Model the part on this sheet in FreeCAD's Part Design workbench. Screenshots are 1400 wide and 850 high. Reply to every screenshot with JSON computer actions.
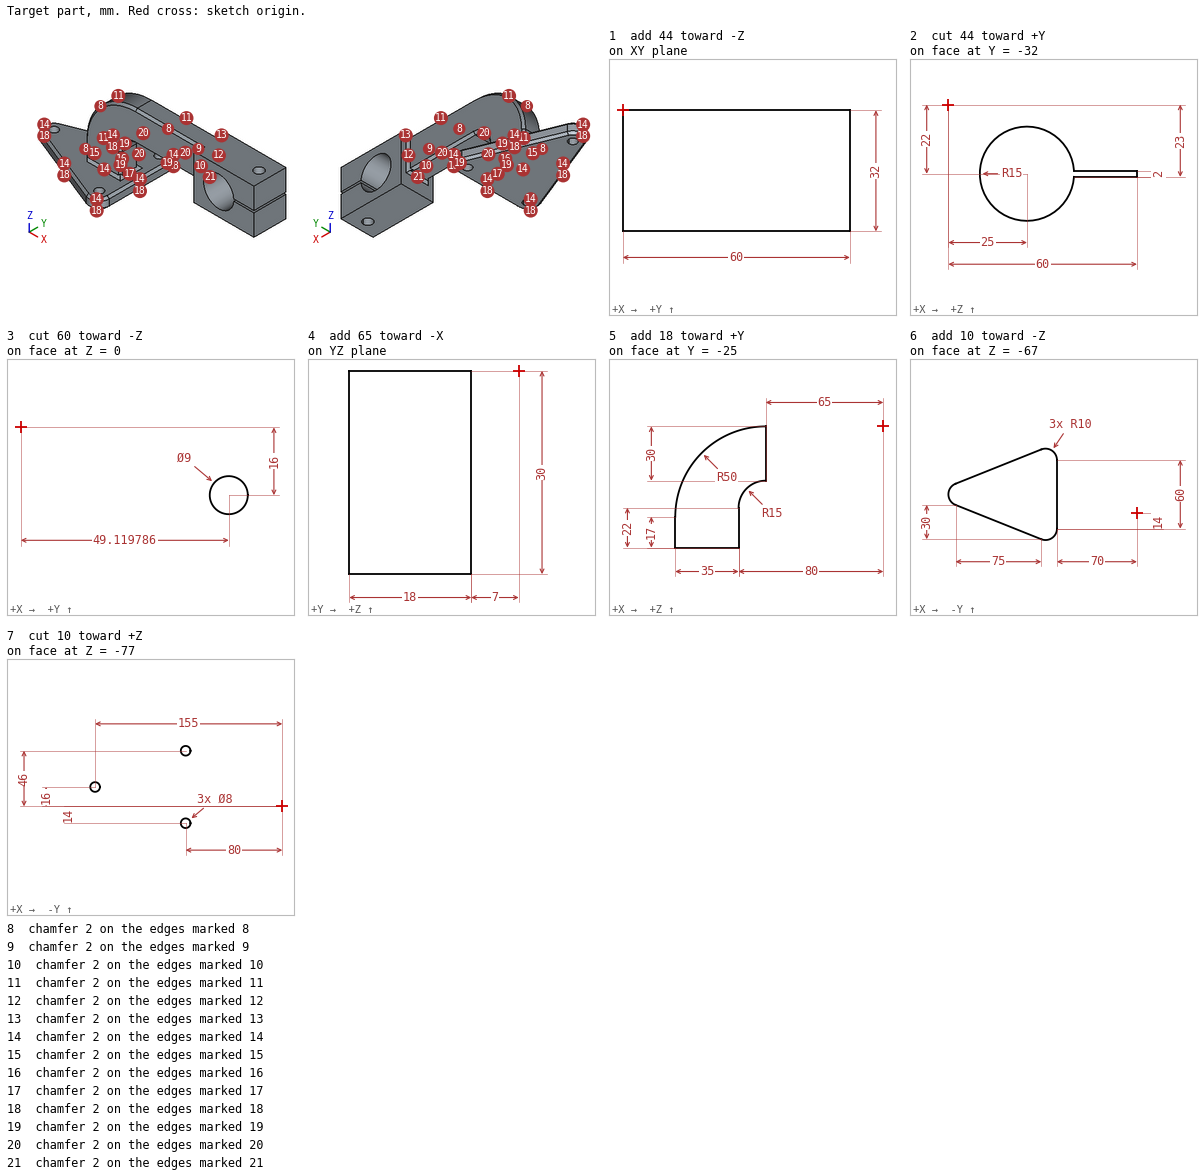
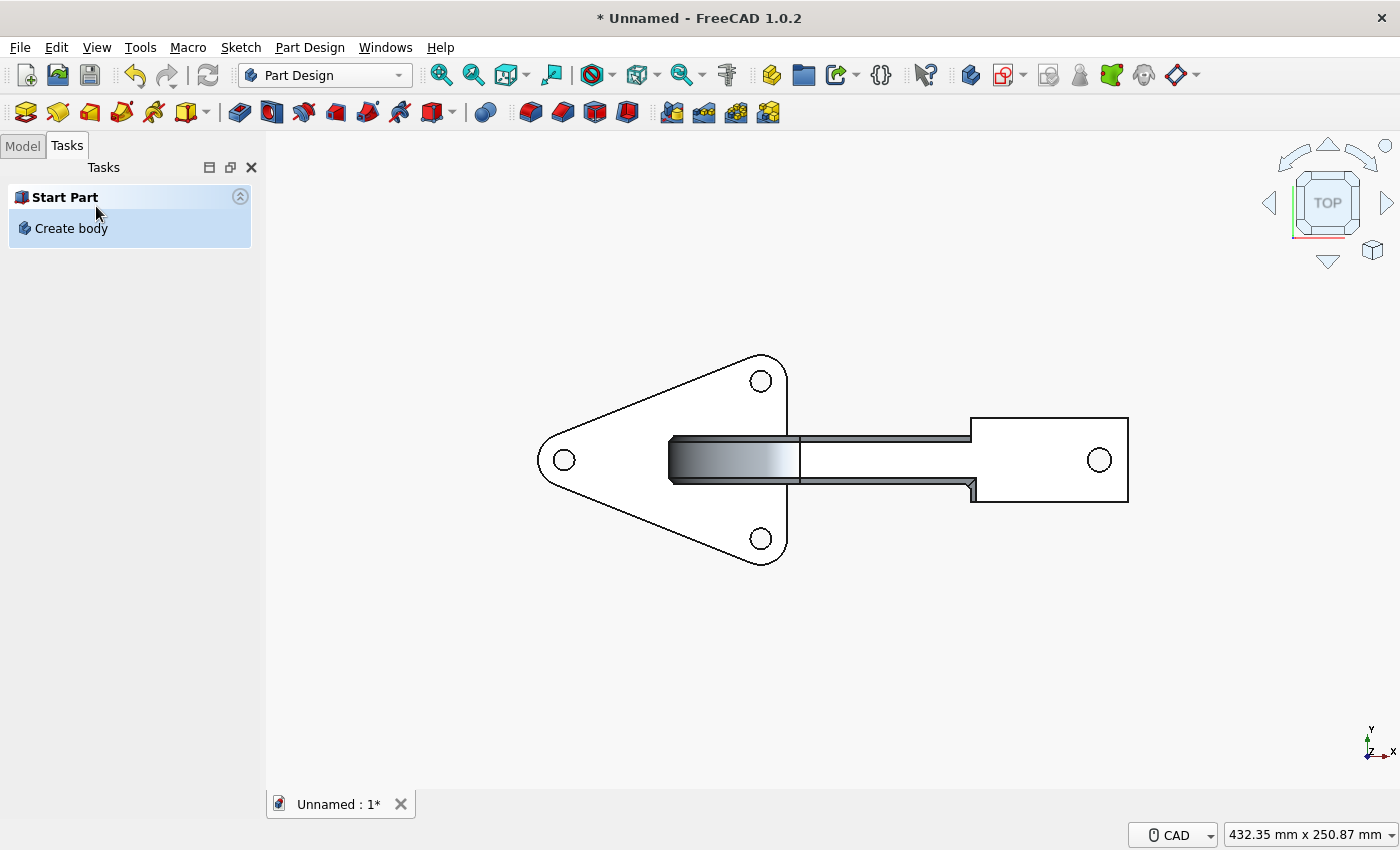
{"action": "key", "text": "1"}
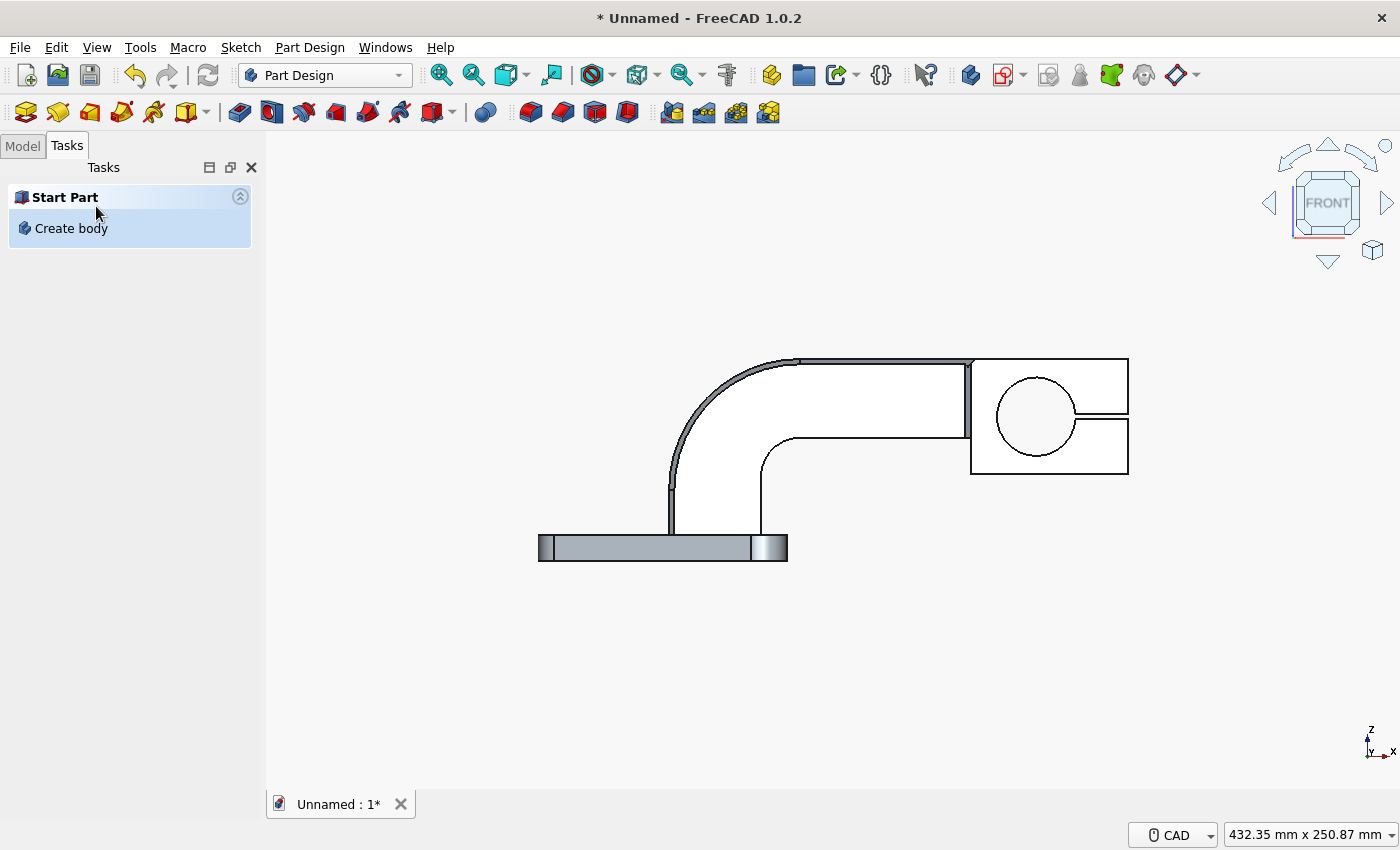
{"action": "key", "text": "3"}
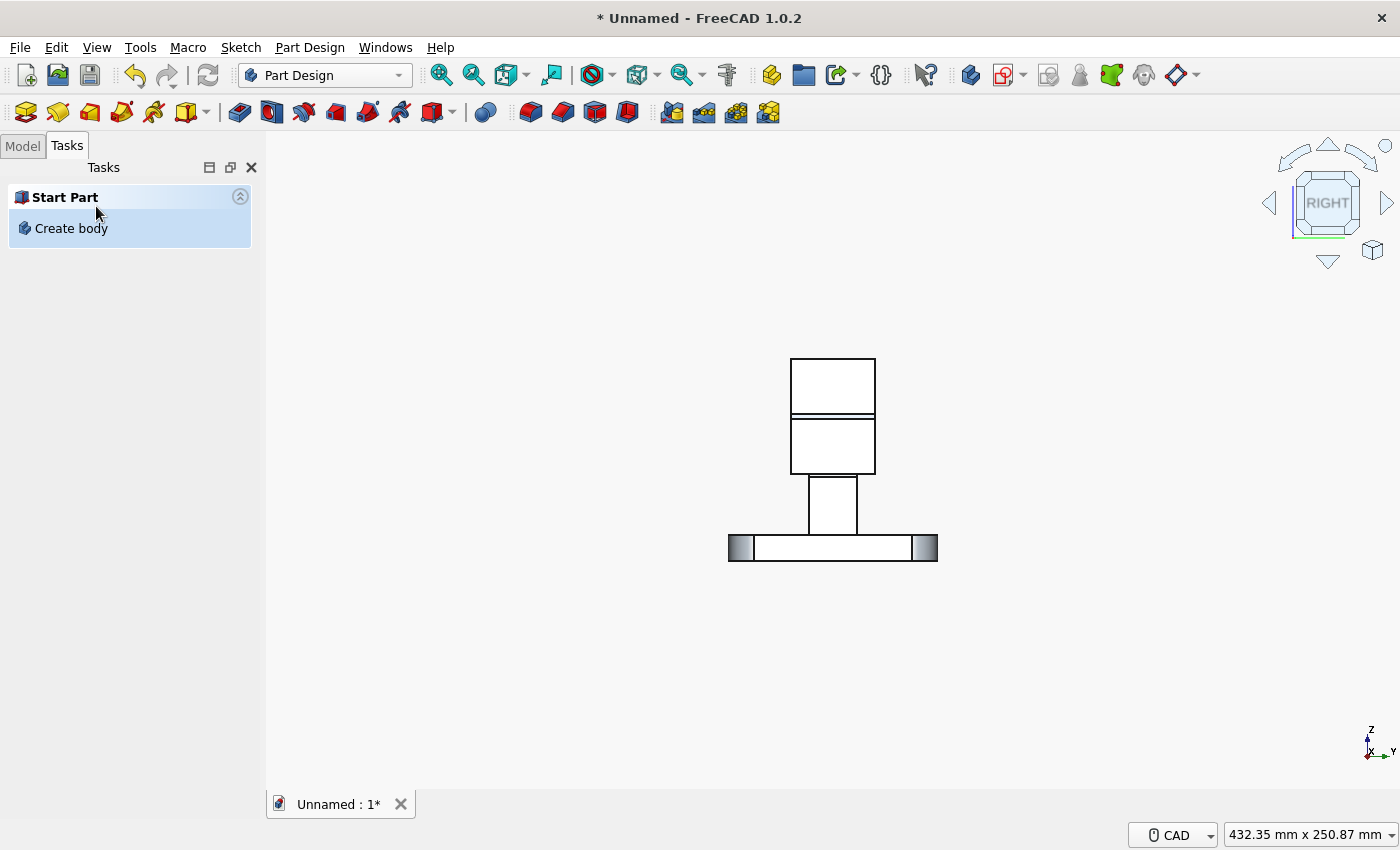
{"action": "left_click", "coordinate": [442, 76]}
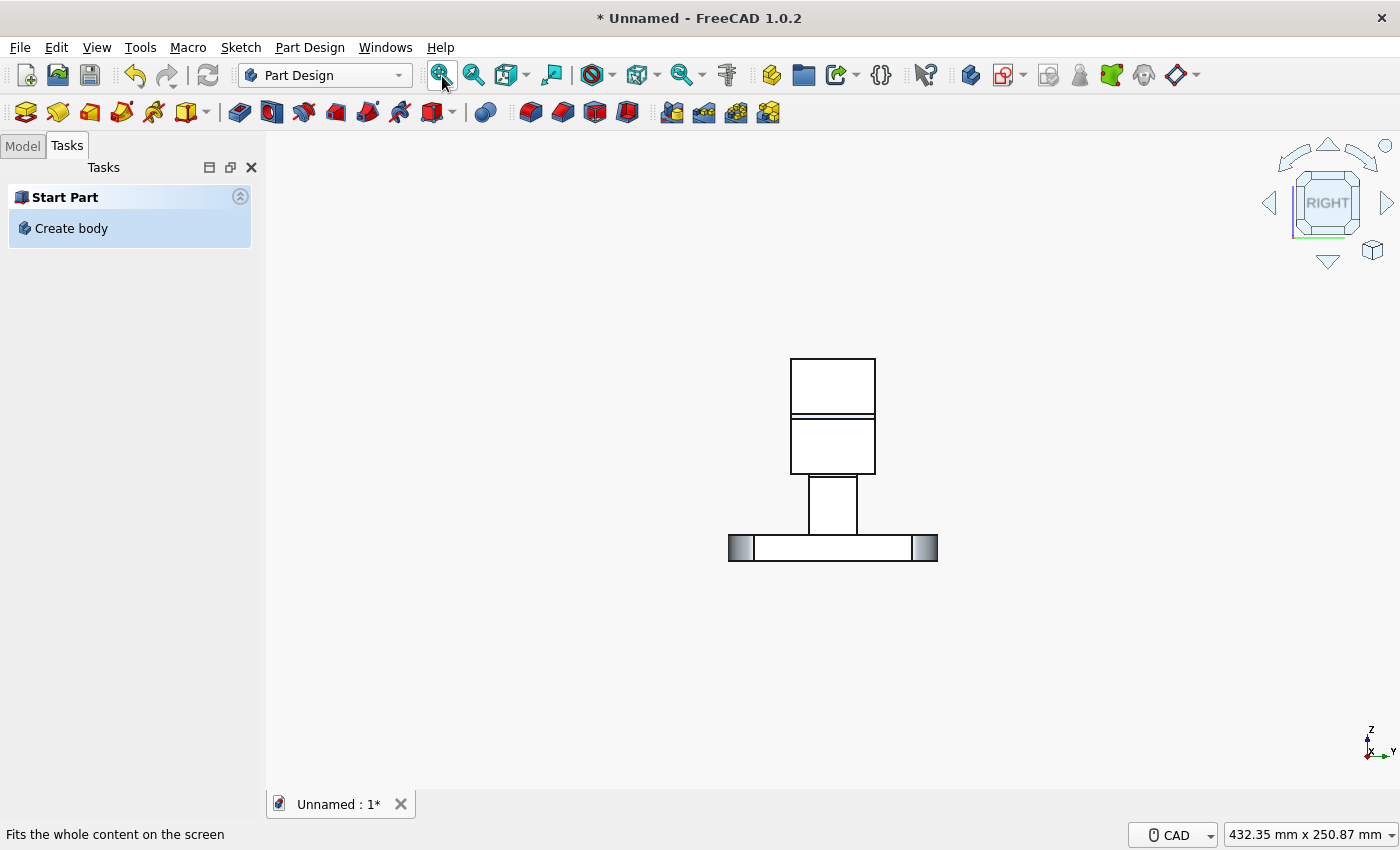
{"action": "key", "text": "5"}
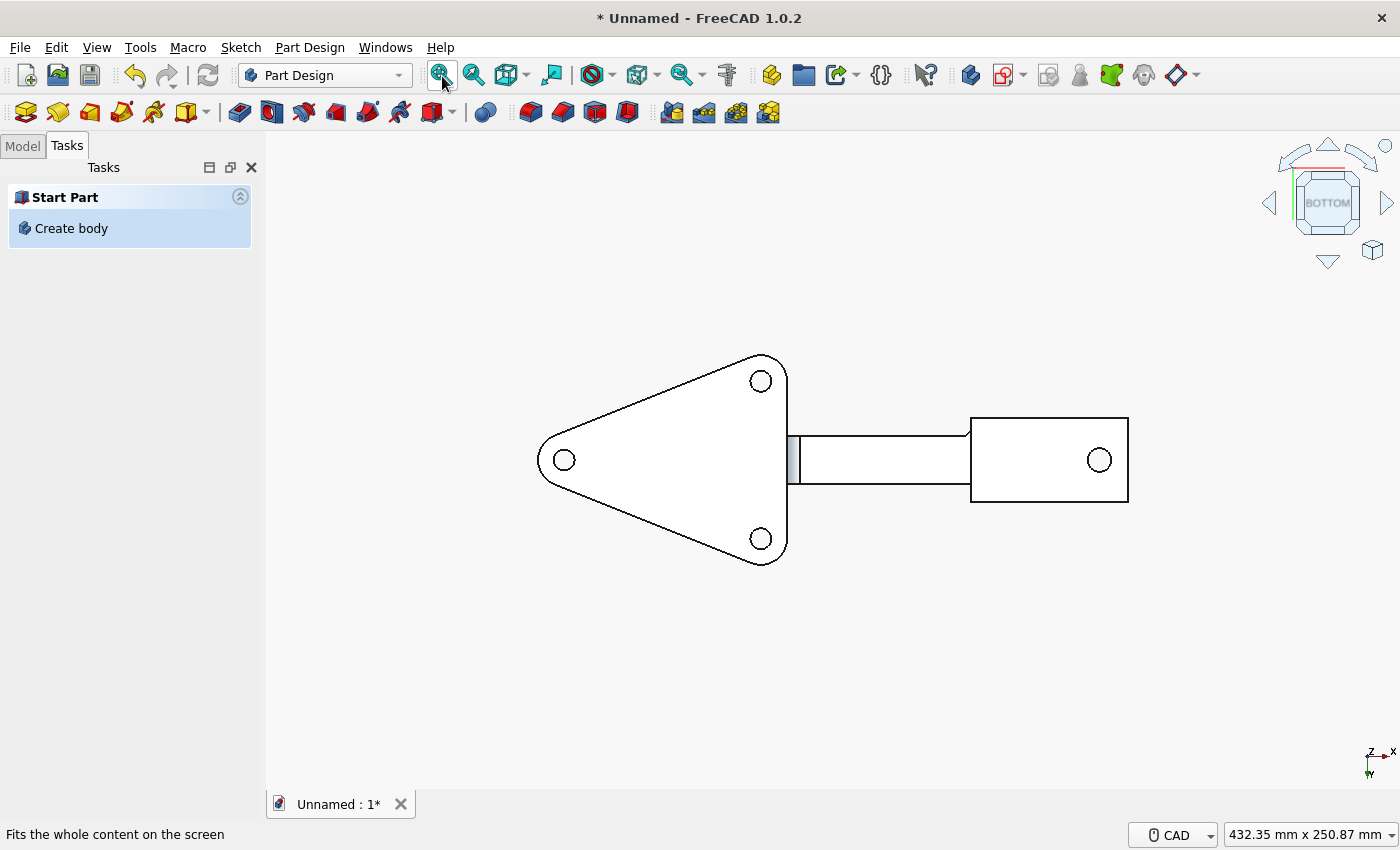
{"action": "key", "text": "4"}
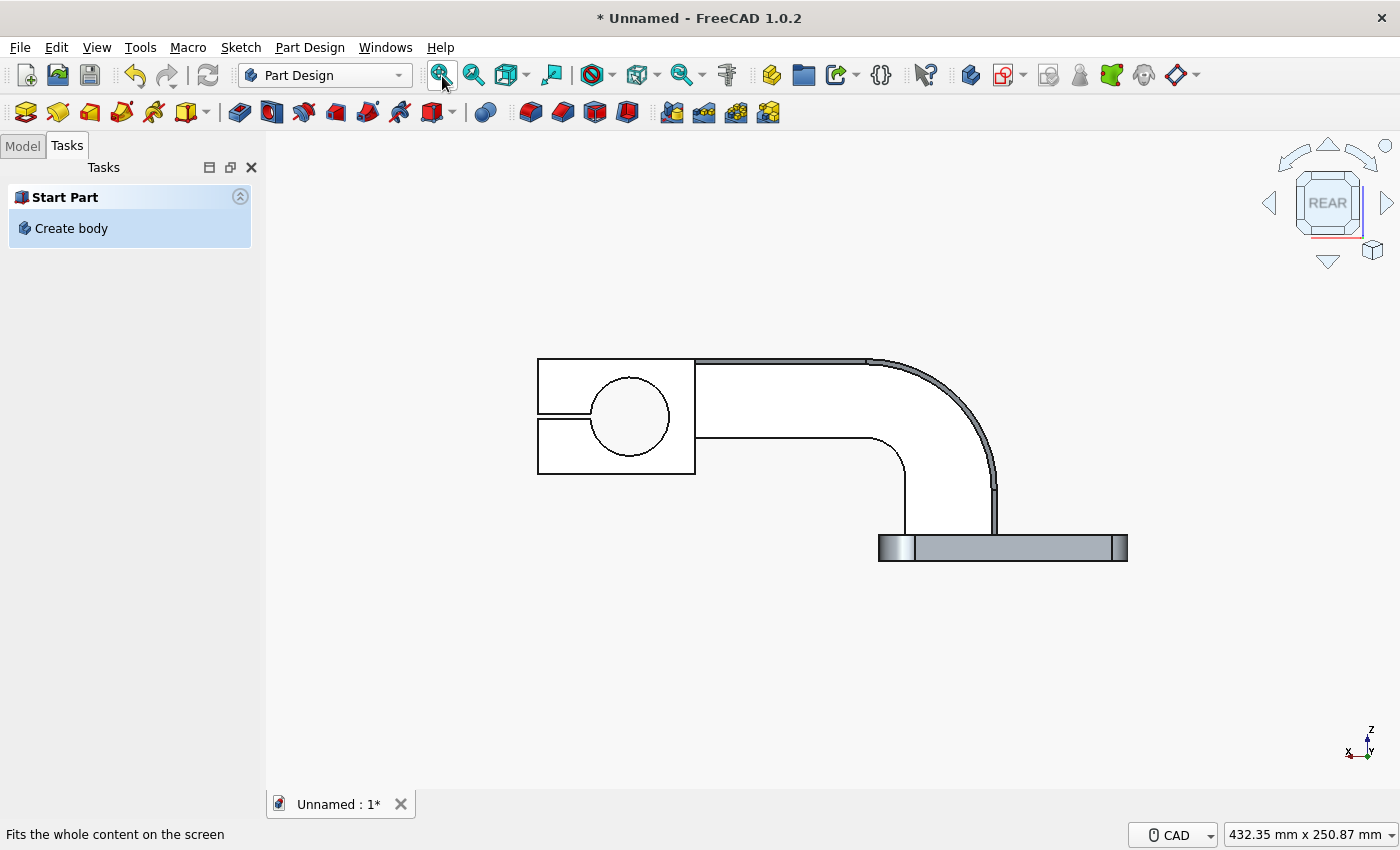
{"action": "key", "text": "6"}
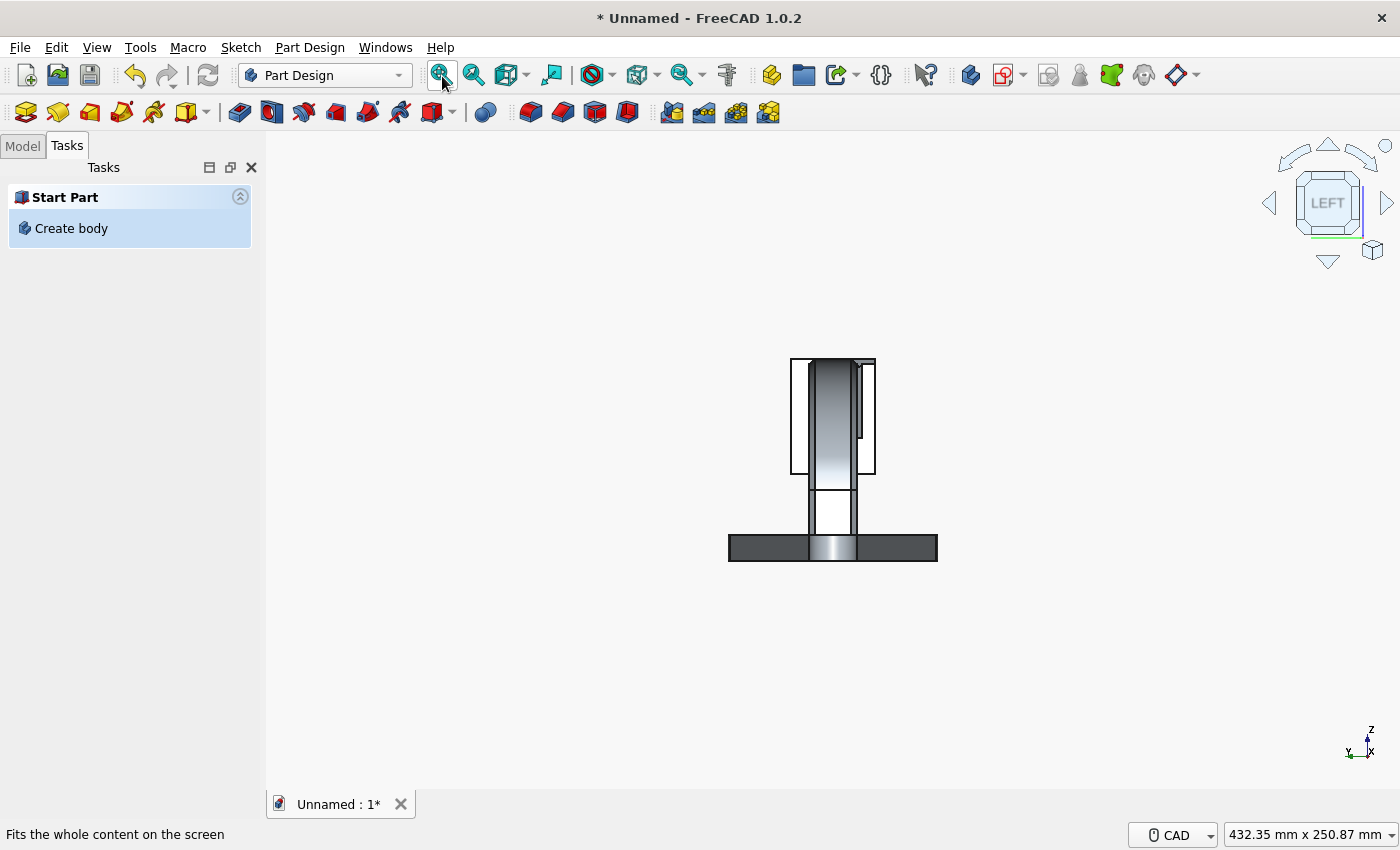
{"action": "left_click", "coordinate": [442, 76]}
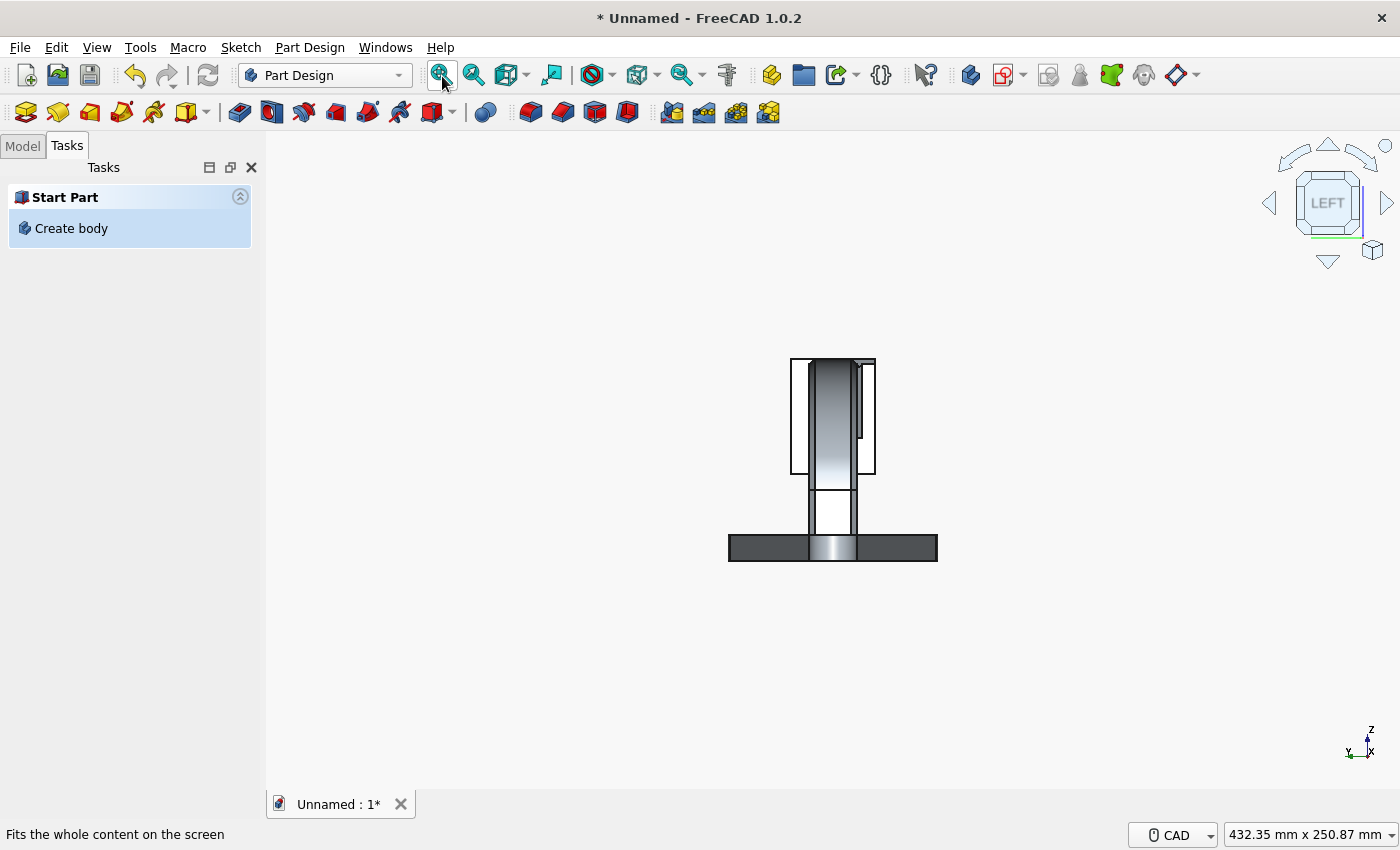
{"action": "key", "text": "v 3"}